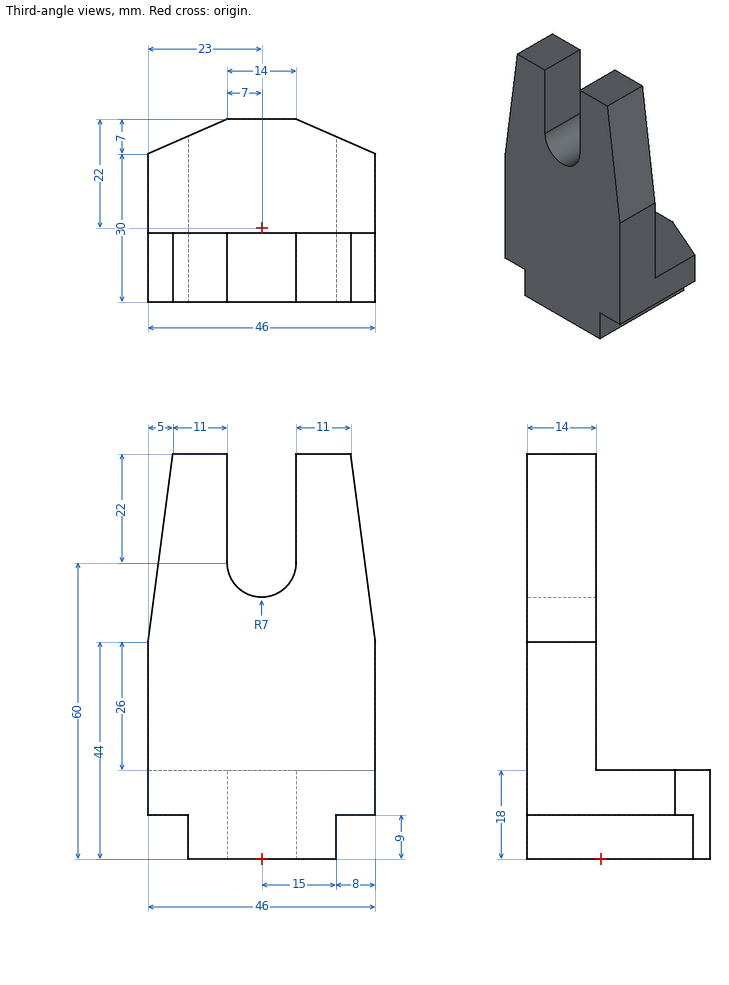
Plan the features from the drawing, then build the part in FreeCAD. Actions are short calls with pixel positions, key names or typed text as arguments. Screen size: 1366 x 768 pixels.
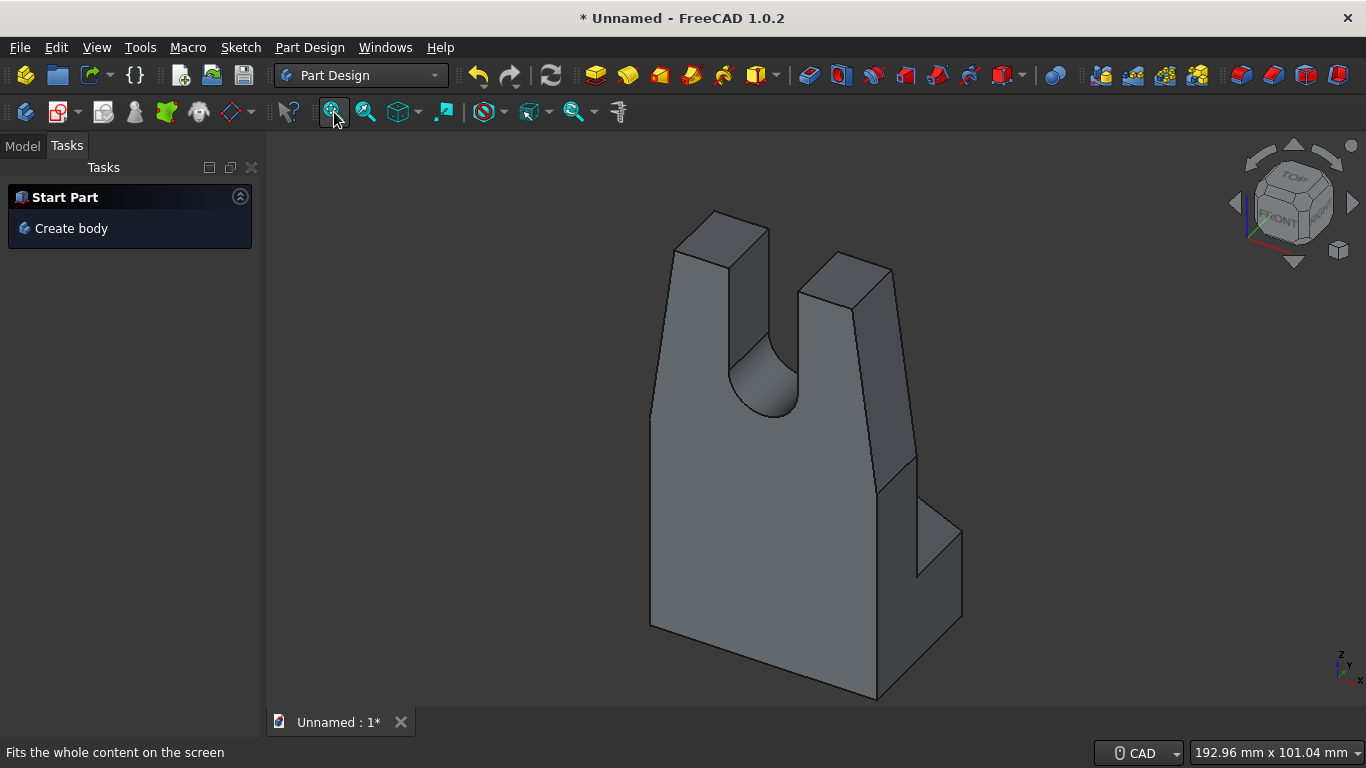
click(763, 525)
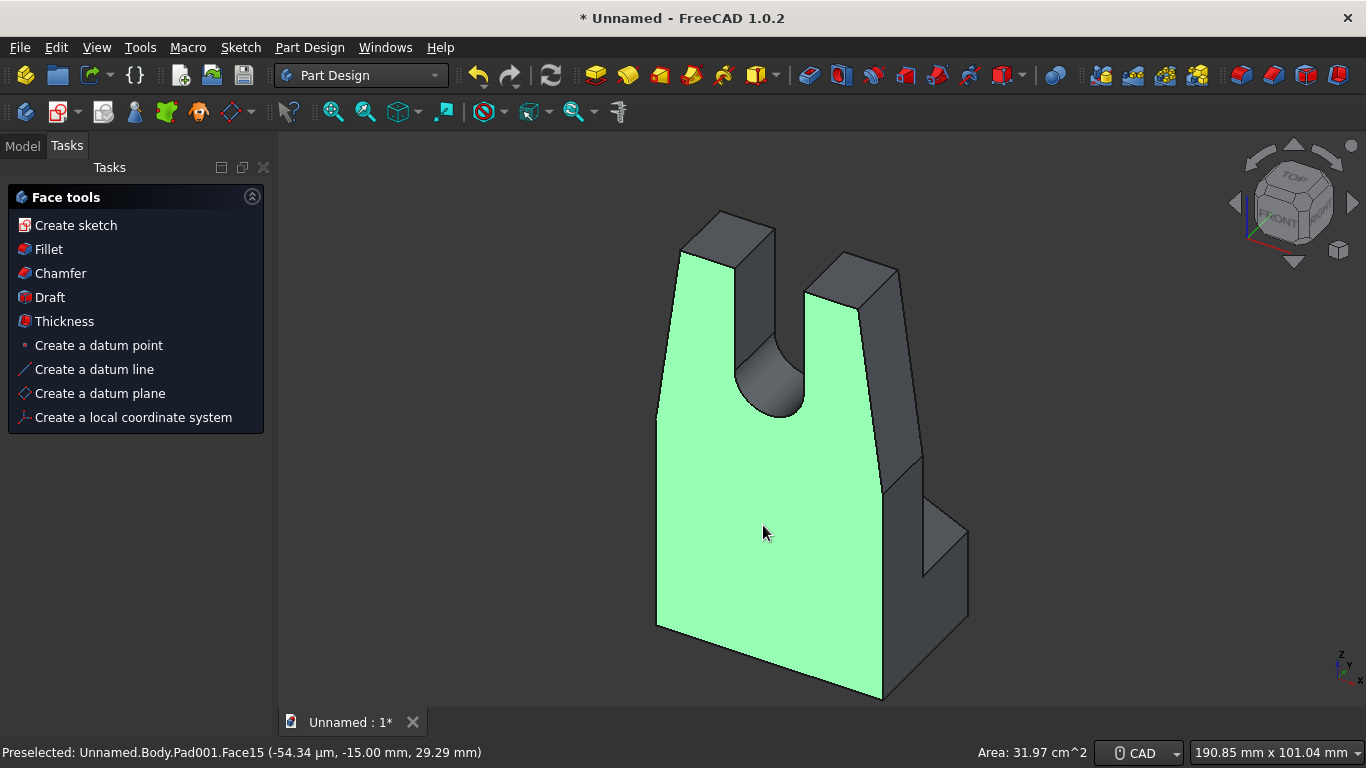
click(58, 112)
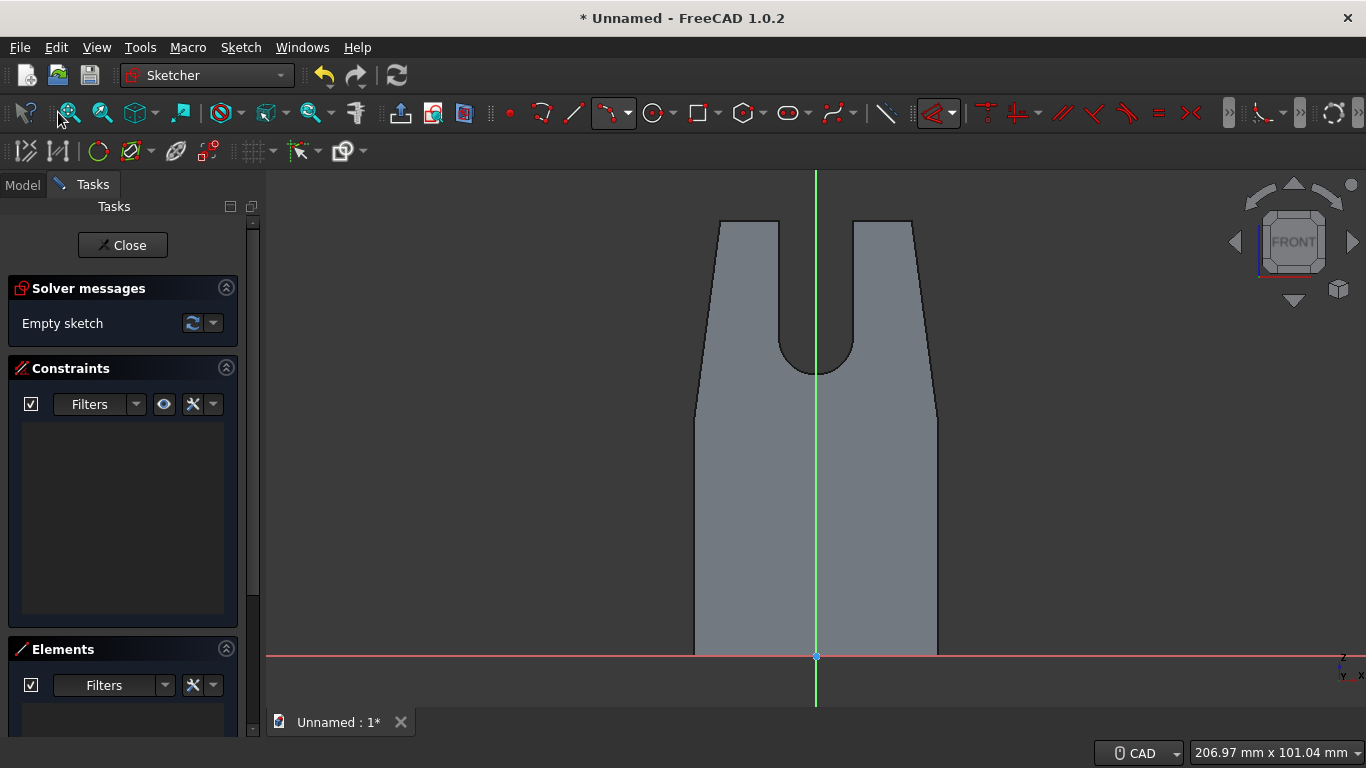
scroll(944, 663, up, 10)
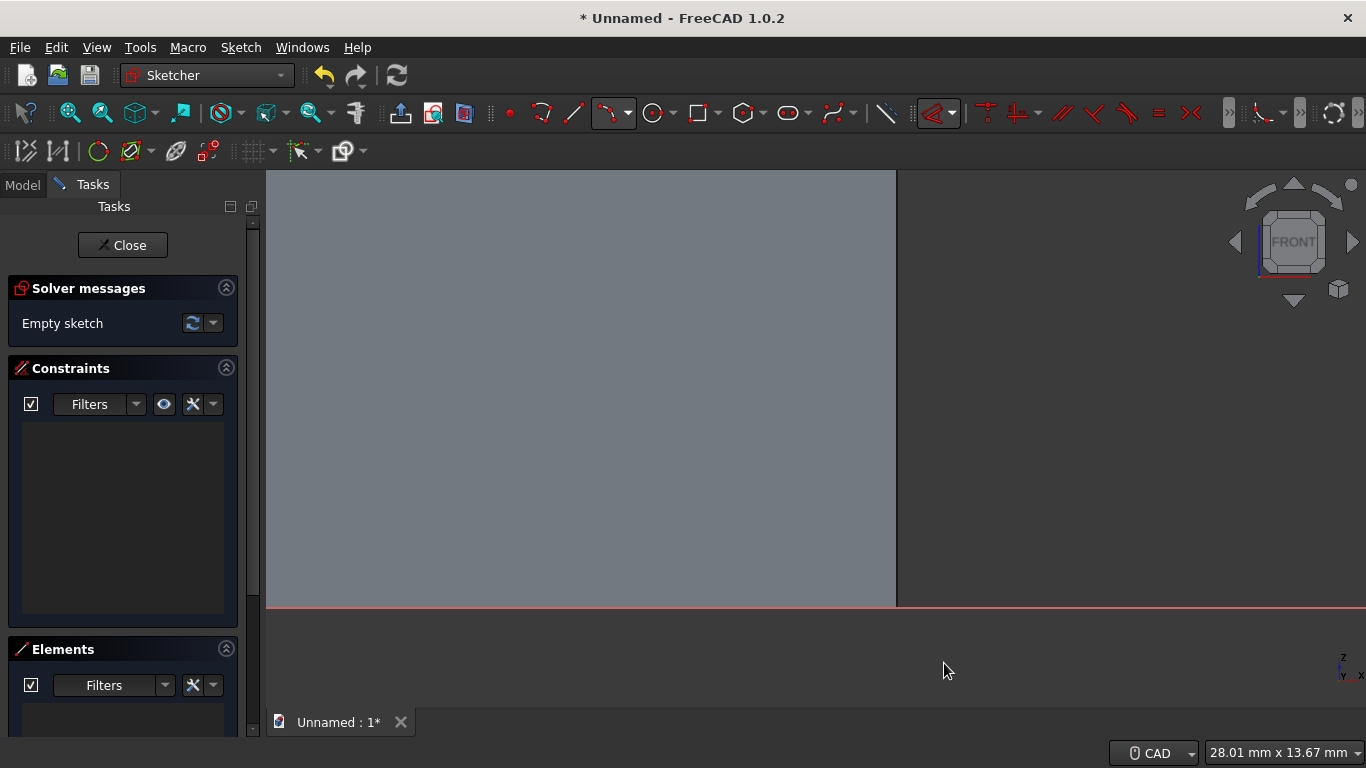
click(698, 114)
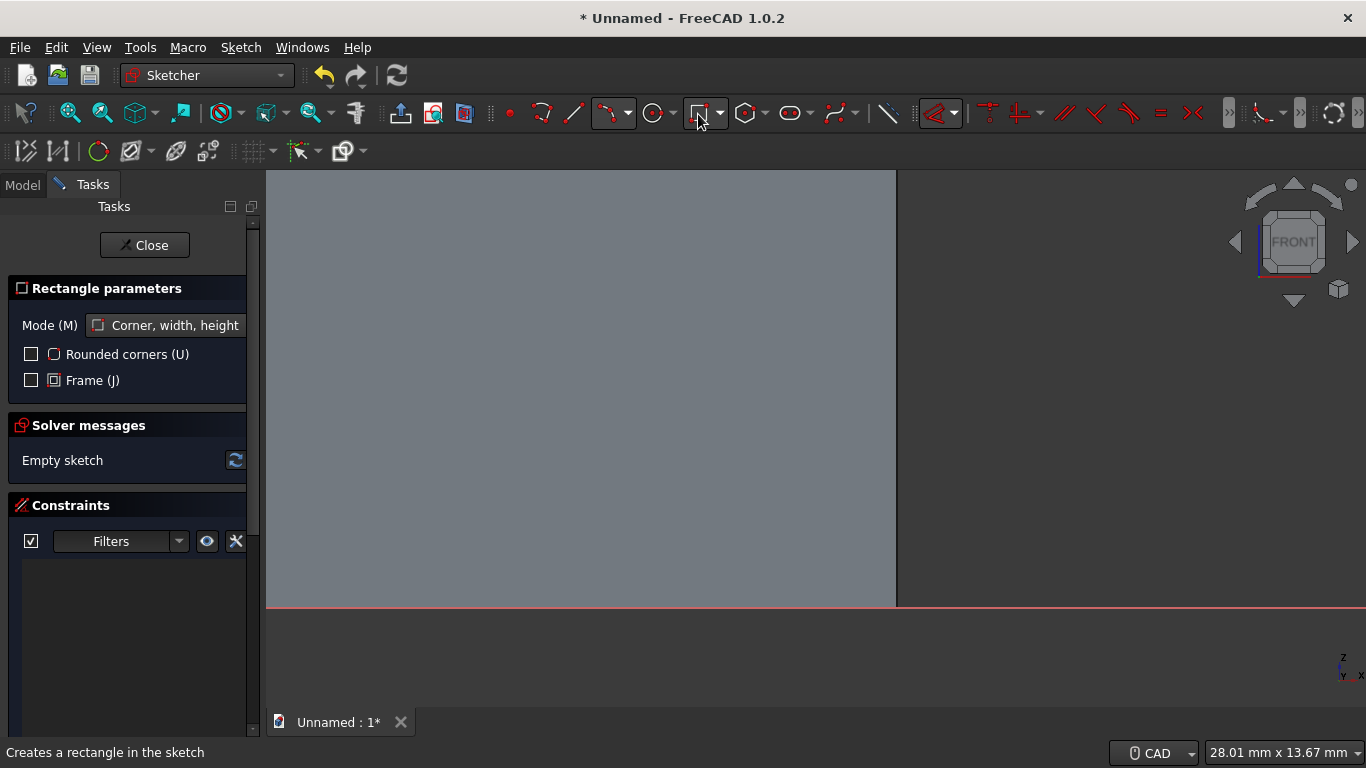
click(583, 255)
click(897, 608)
key(Escape)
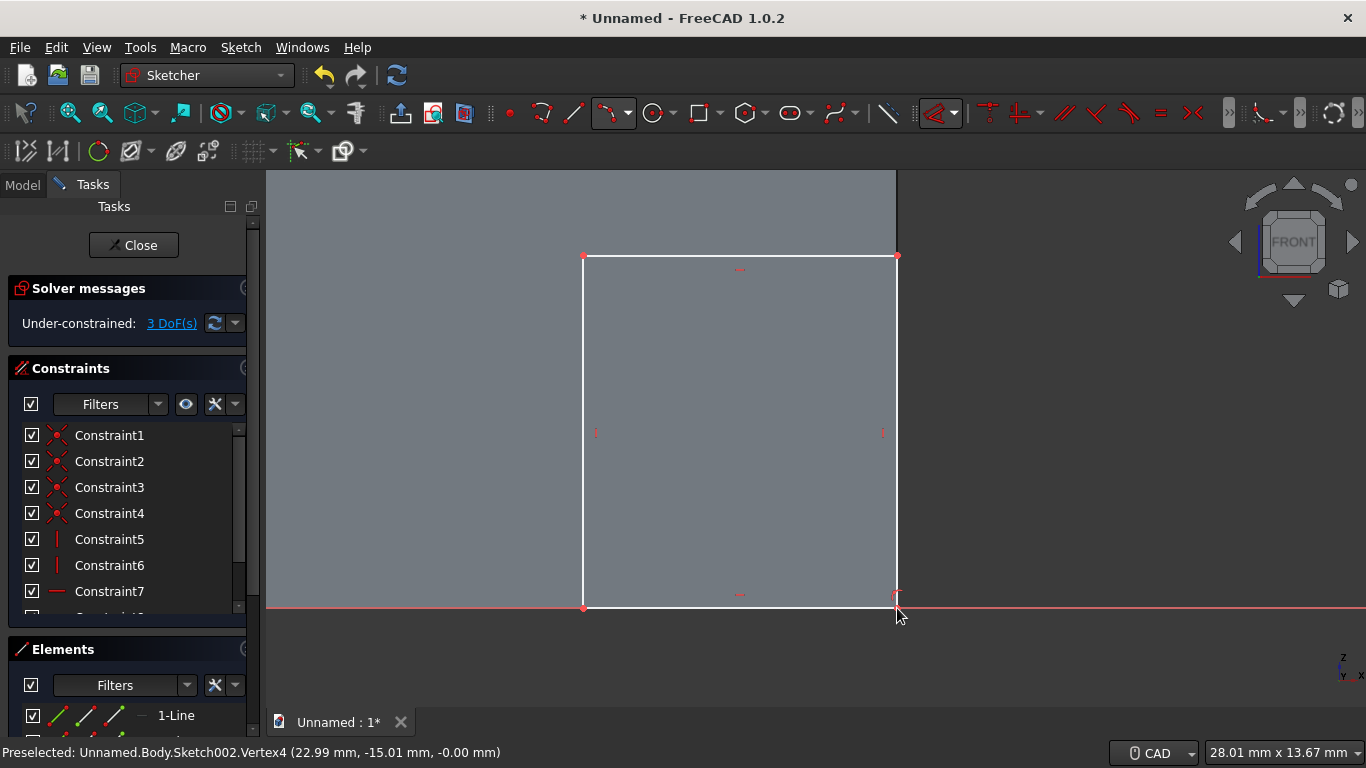
click(583, 362)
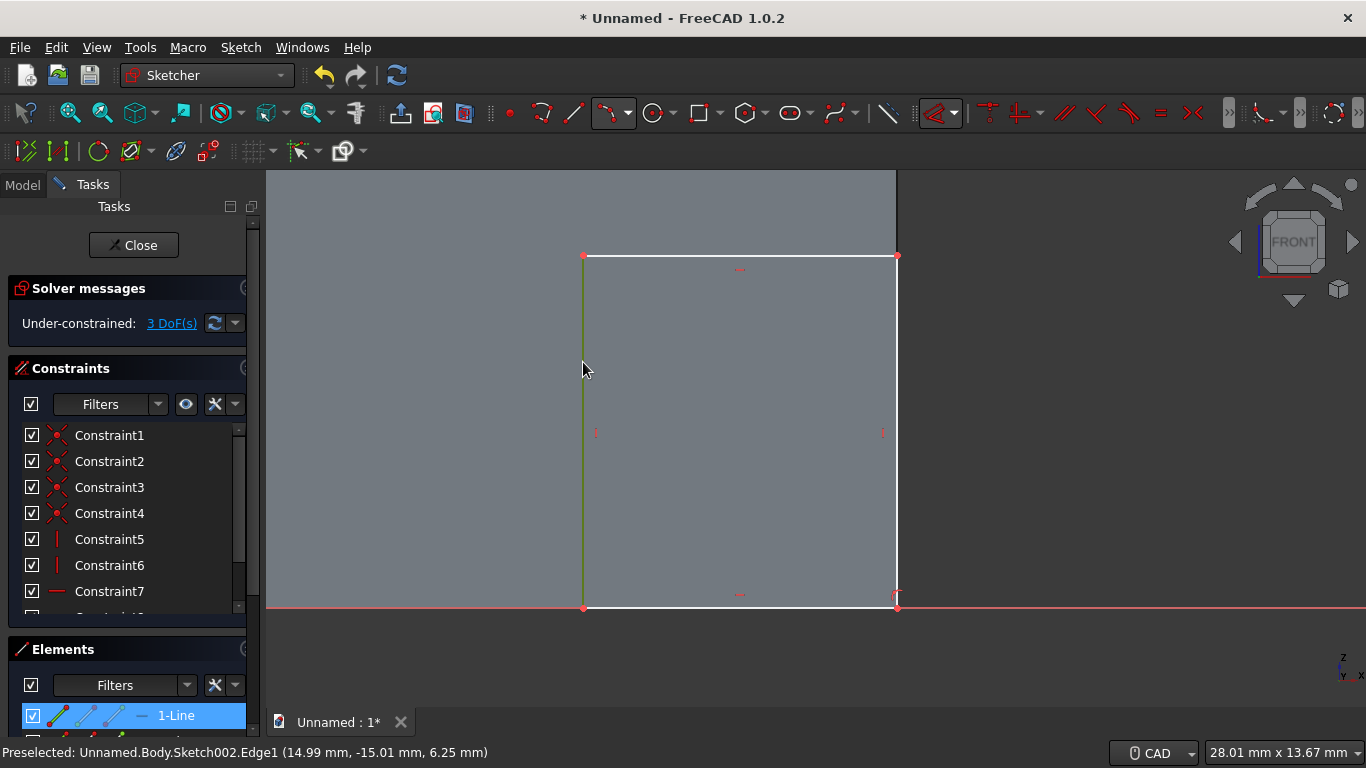
click(956, 114)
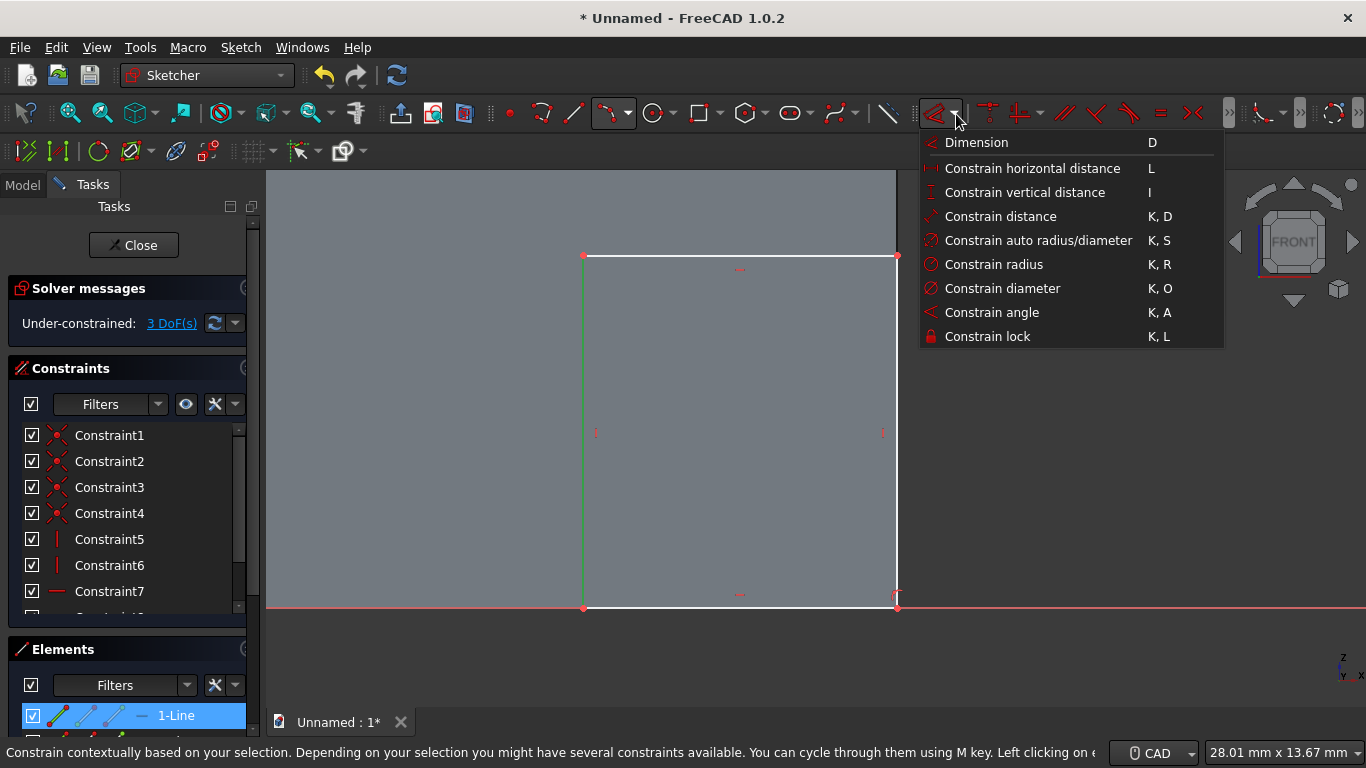
click(1072, 192)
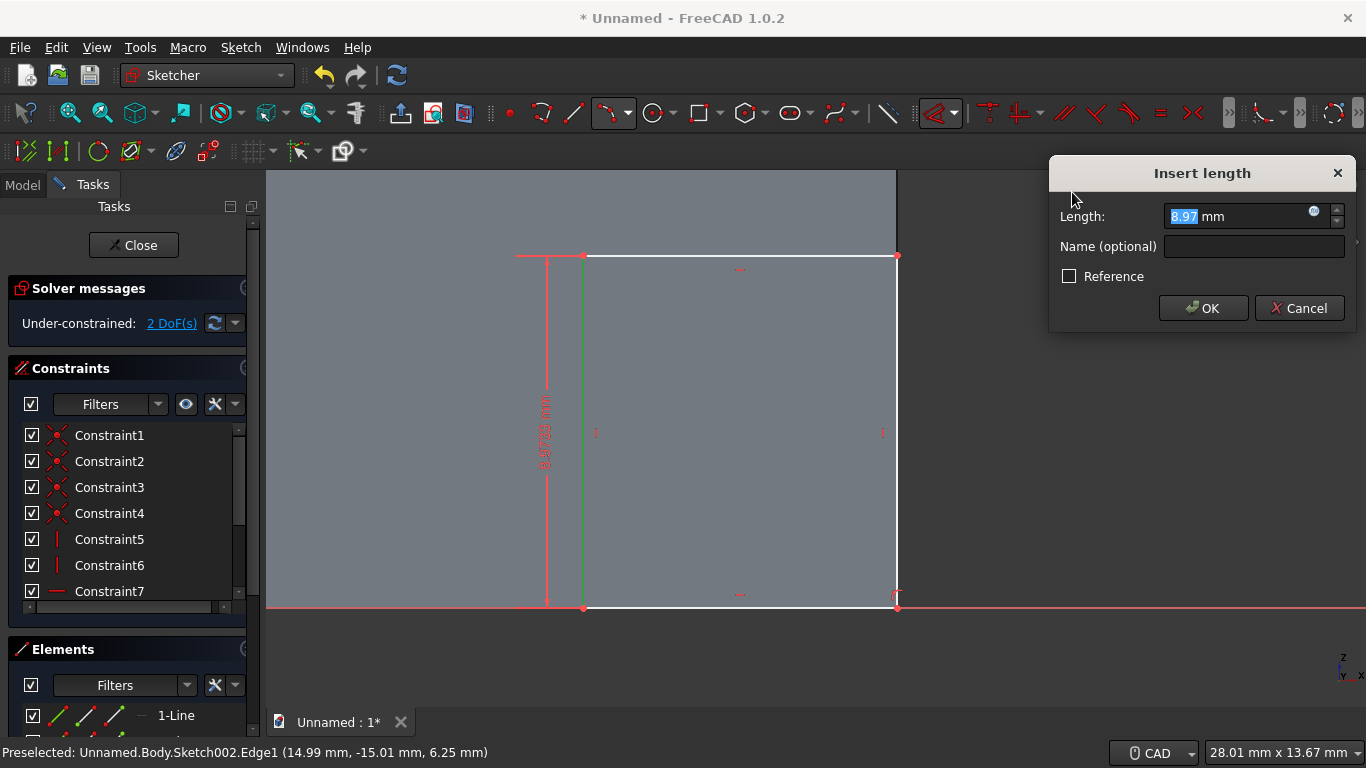
text(9)
key(Return)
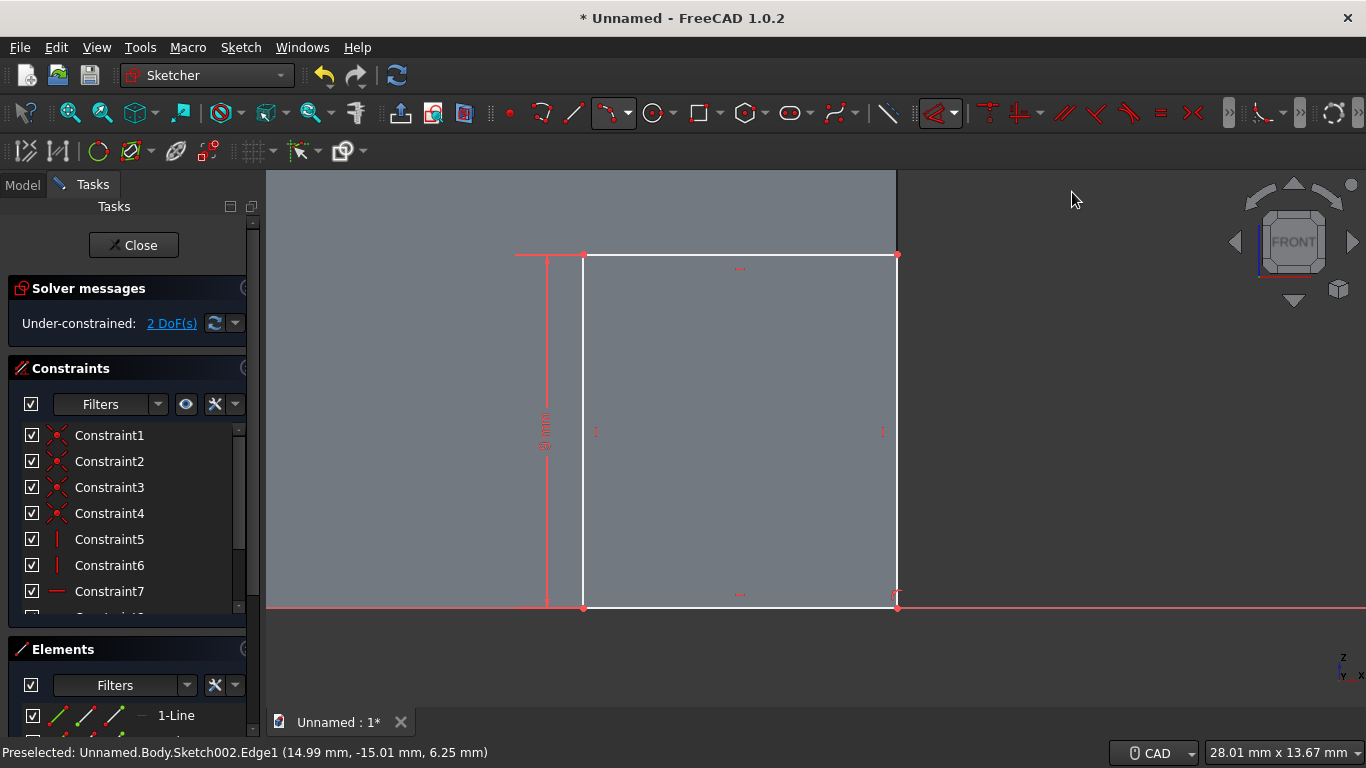
click(677, 608)